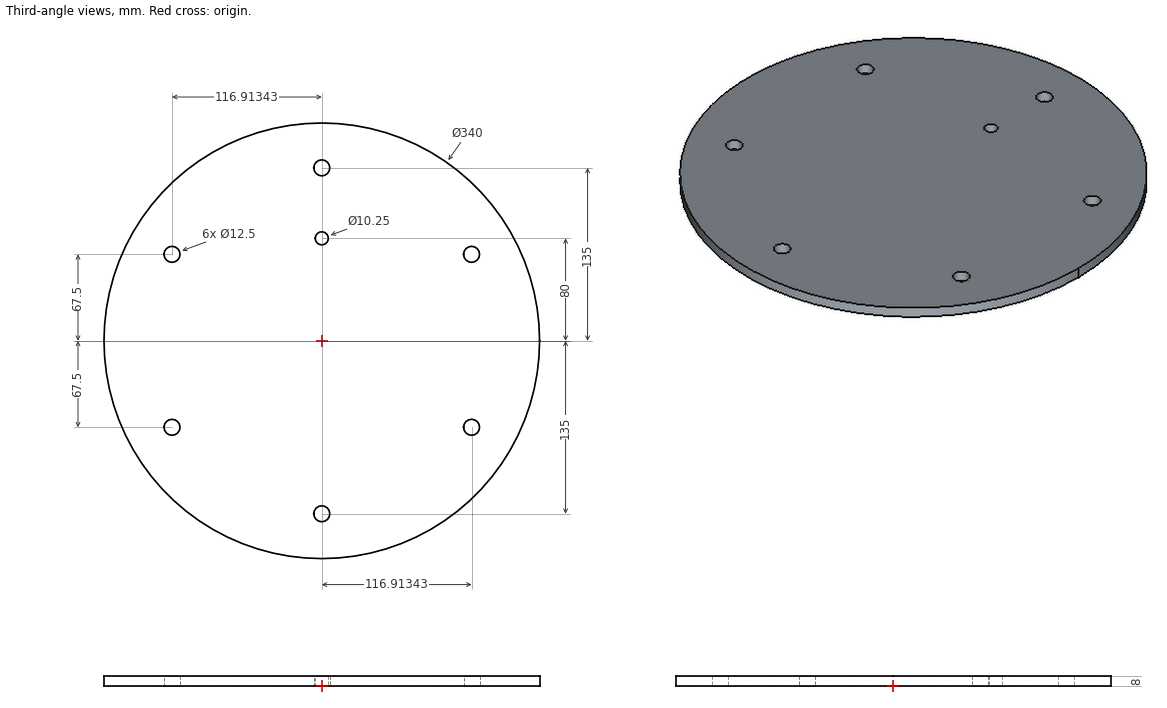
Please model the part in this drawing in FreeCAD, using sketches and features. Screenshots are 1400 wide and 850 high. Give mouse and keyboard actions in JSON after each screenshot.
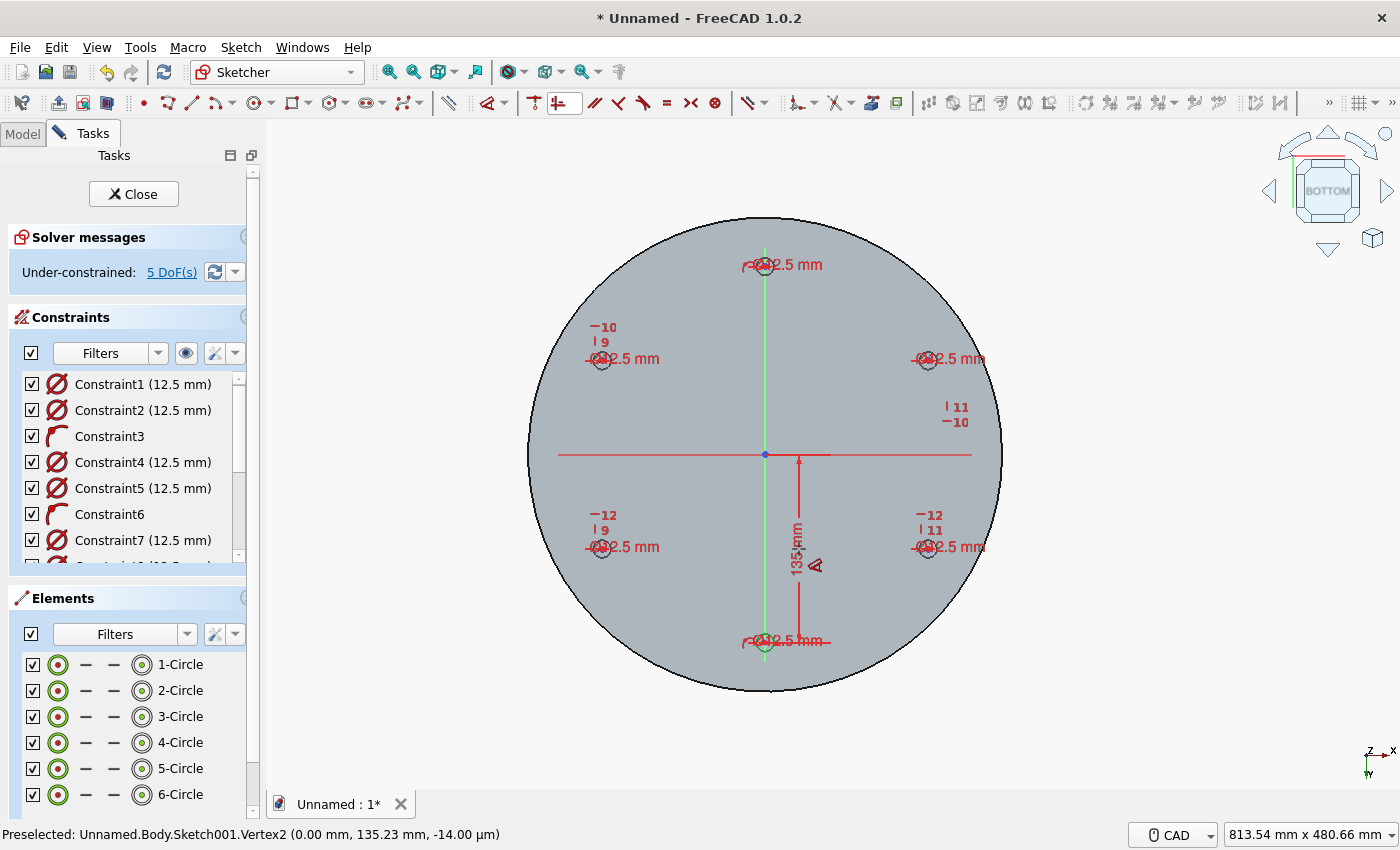
{"action": "left_click", "coordinate": [765, 267]}
{"action": "left_click", "coordinate": [799, 361]}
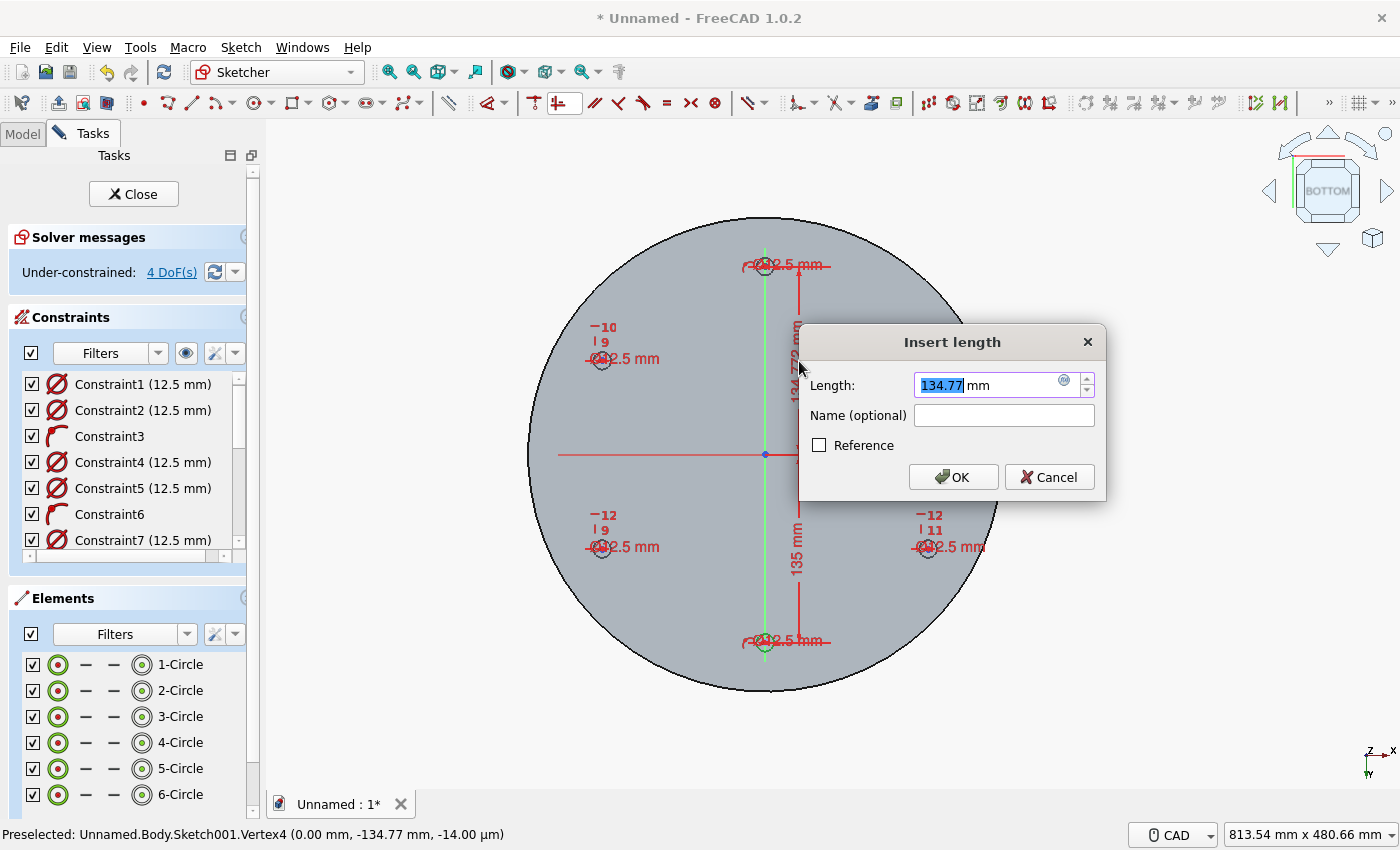
{"action": "type", "text": "135"}
{"action": "key", "text": "Return"}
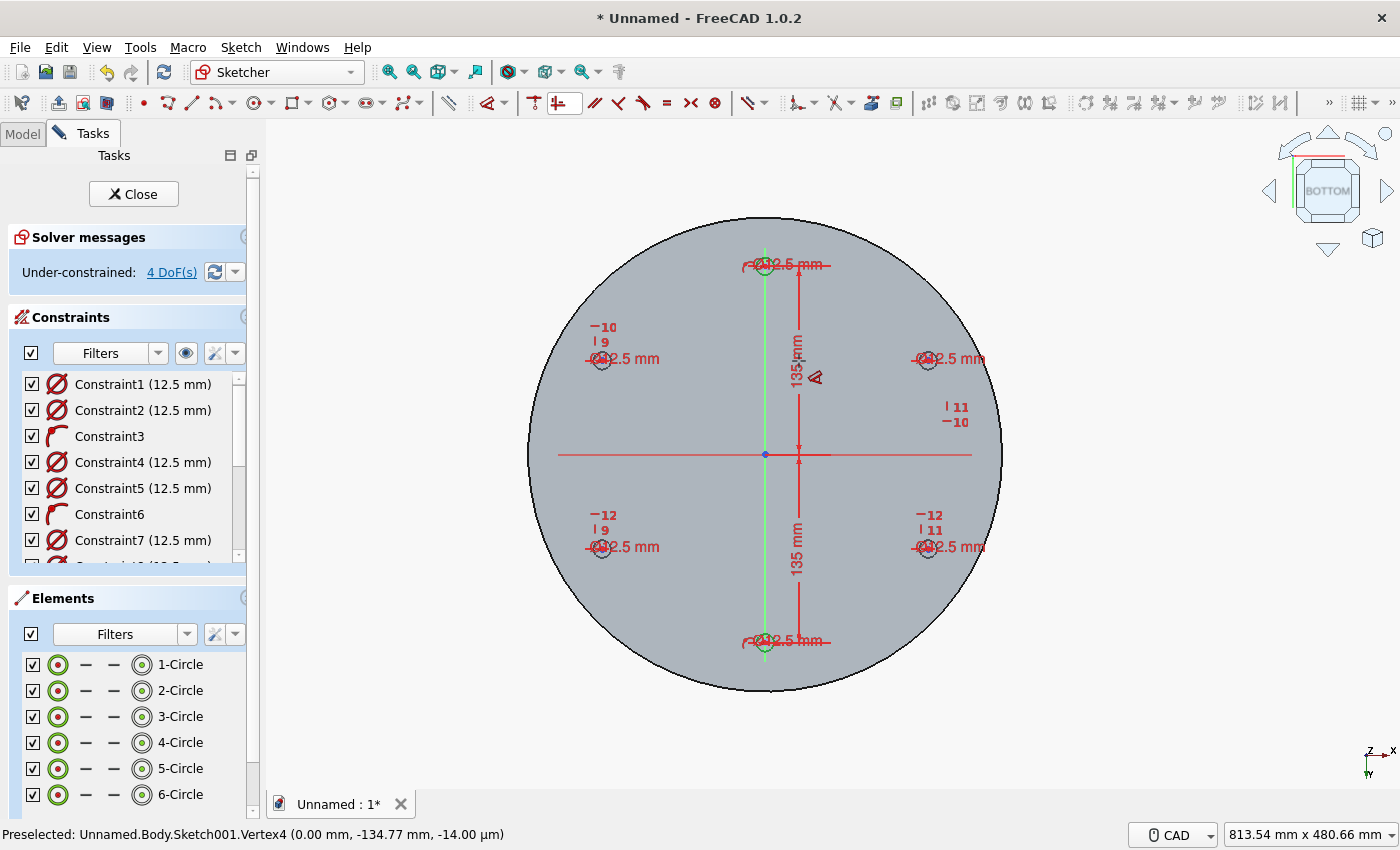
{"action": "left_click", "coordinate": [602, 549]}
{"action": "left_click", "coordinate": [568, 502]}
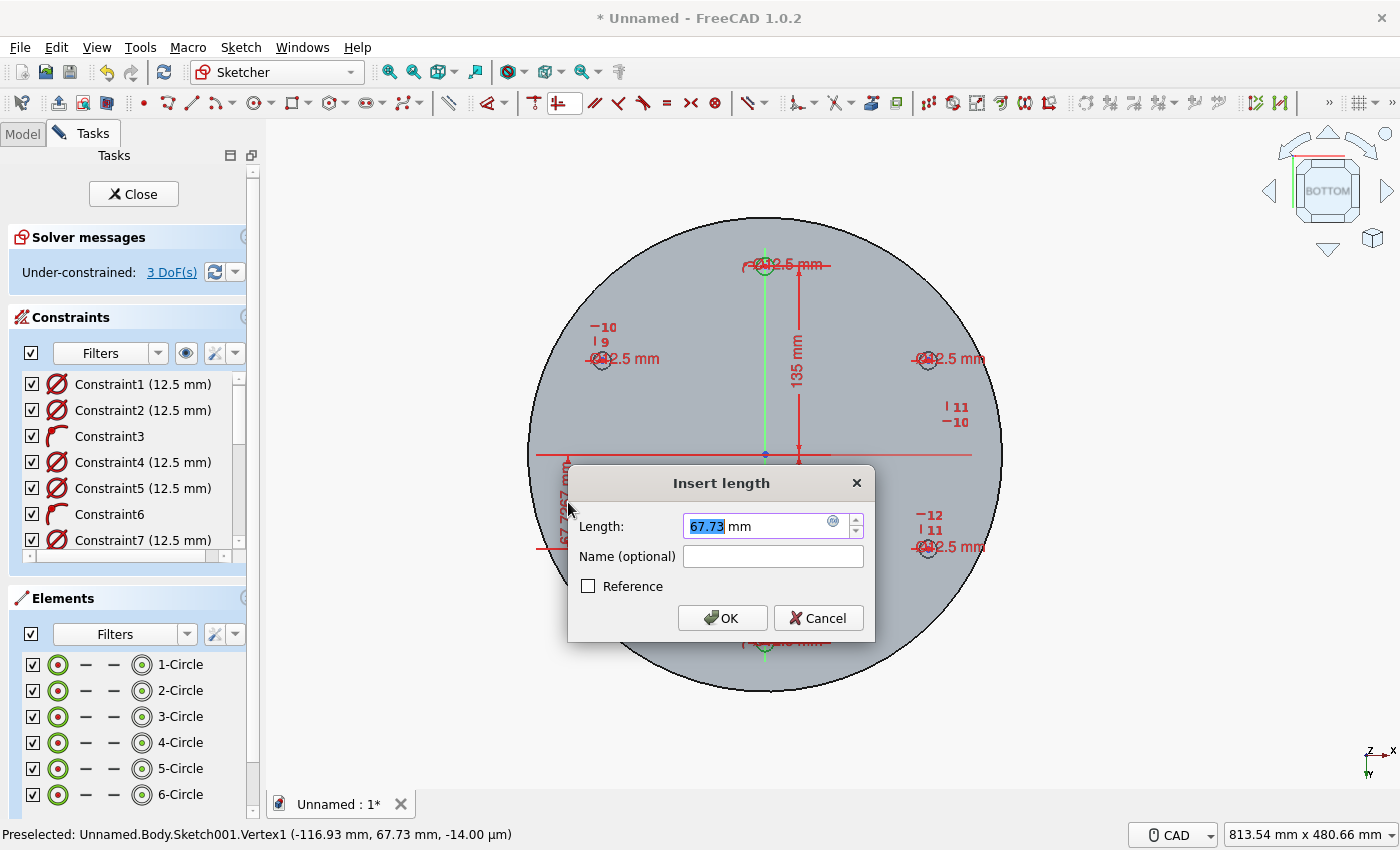
{"action": "type", "text": "67.5"}
{"action": "key", "text": "Return"}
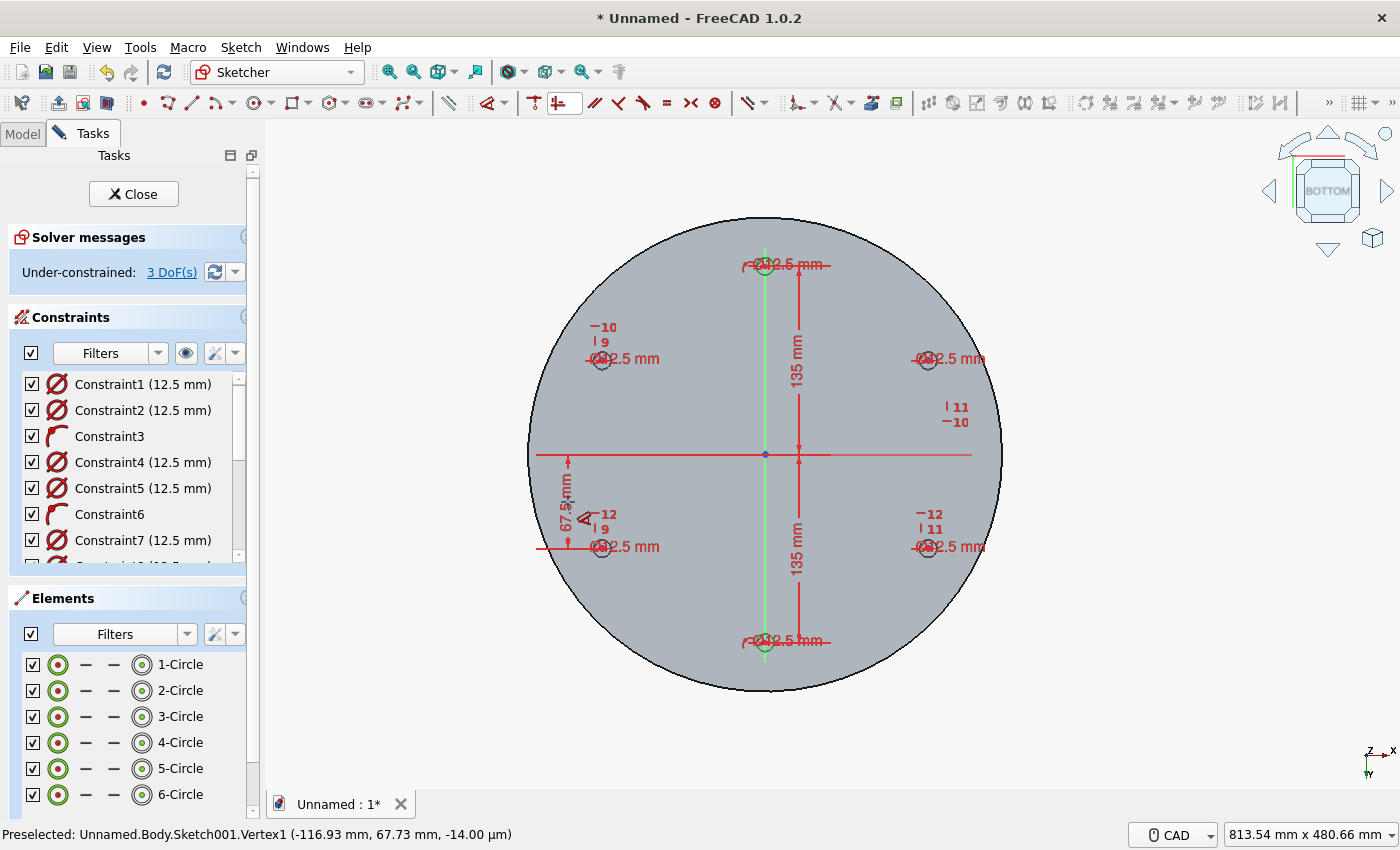
{"action": "left_click", "coordinate": [602, 361]}
{"action": "left_click", "coordinate": [568, 408]}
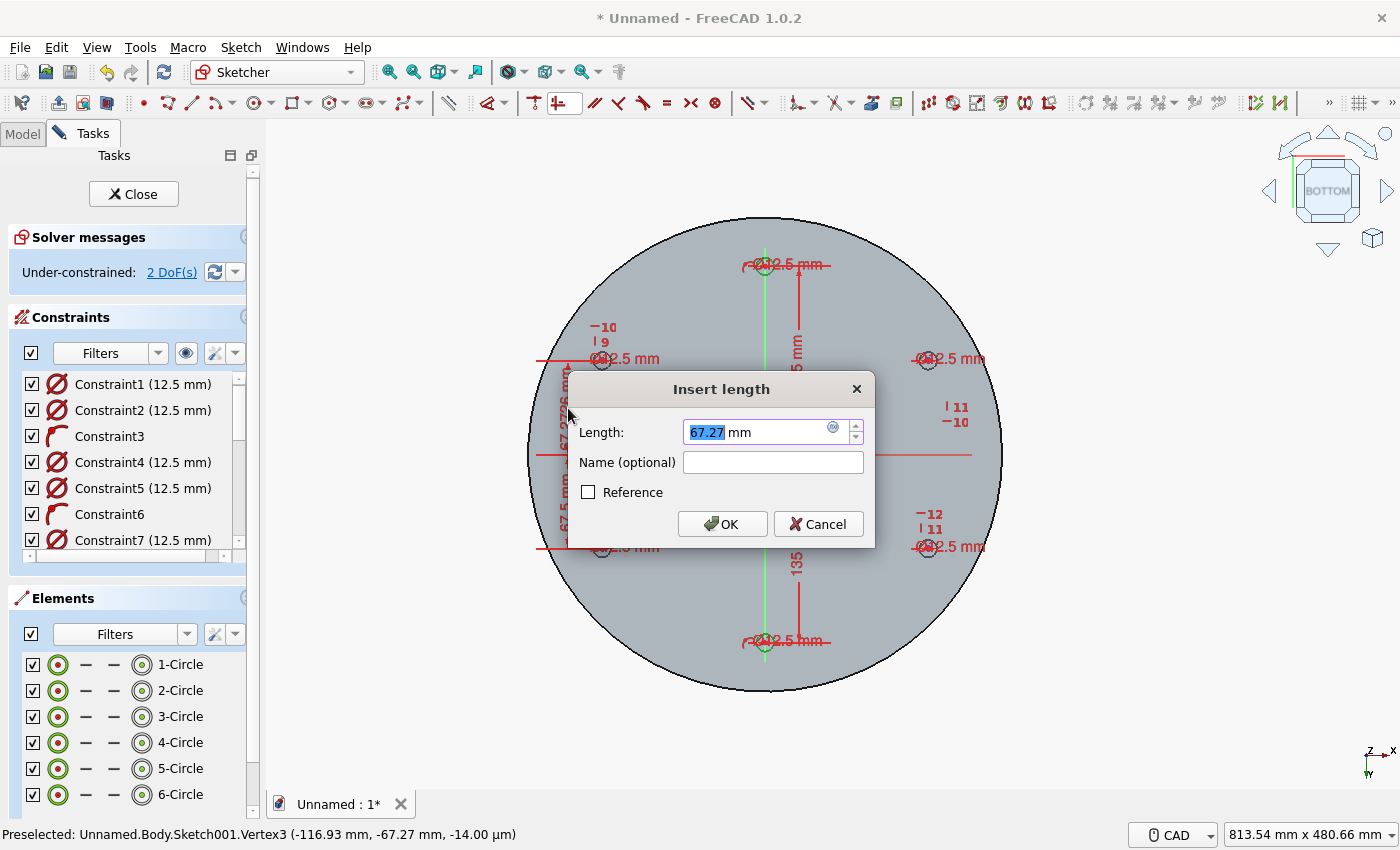
{"action": "type", "text": "67.5"}
{"action": "key", "text": "Return"}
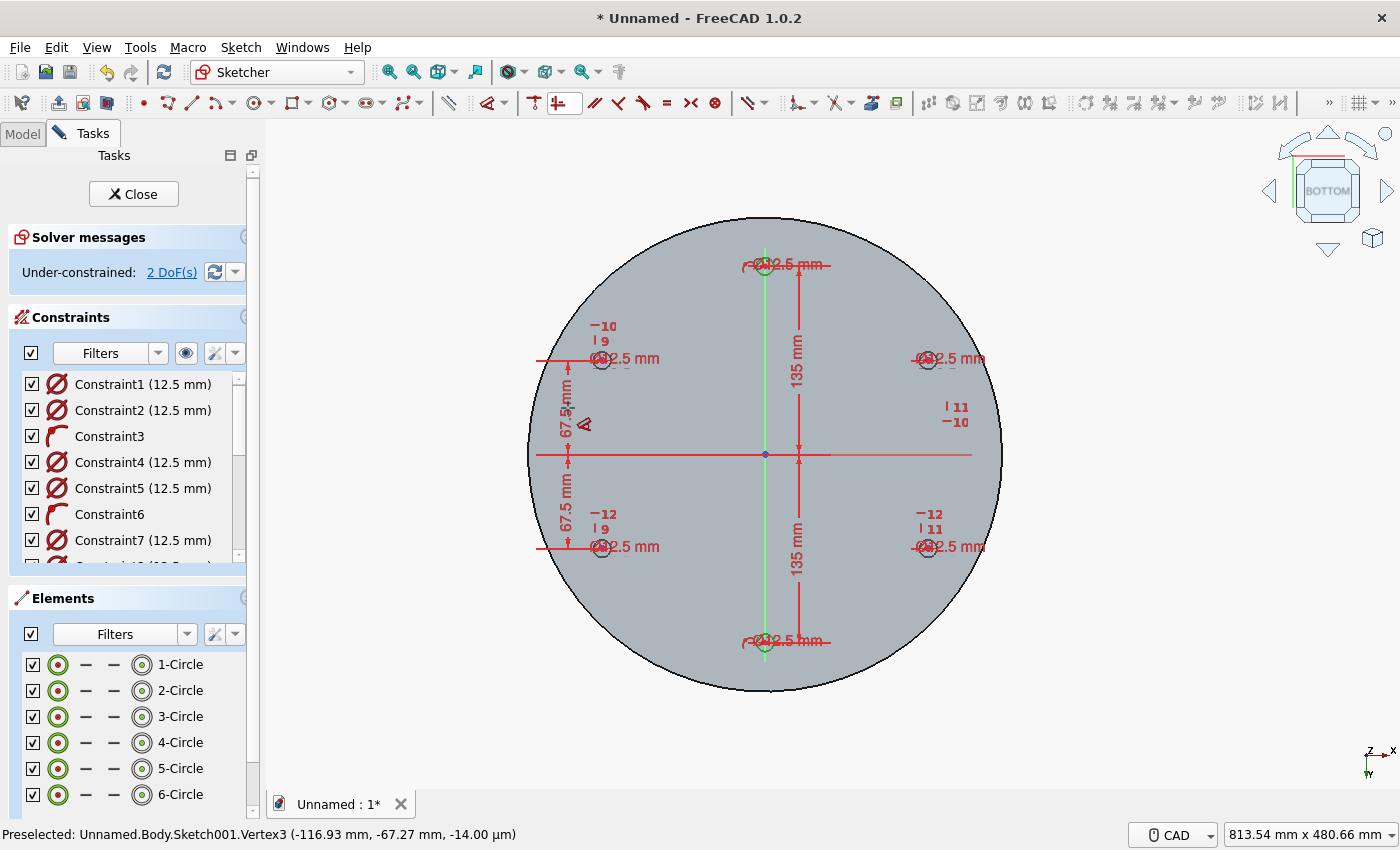
{"action": "left_click", "coordinate": [602, 549]}
{"action": "left_click", "coordinate": [684, 583]}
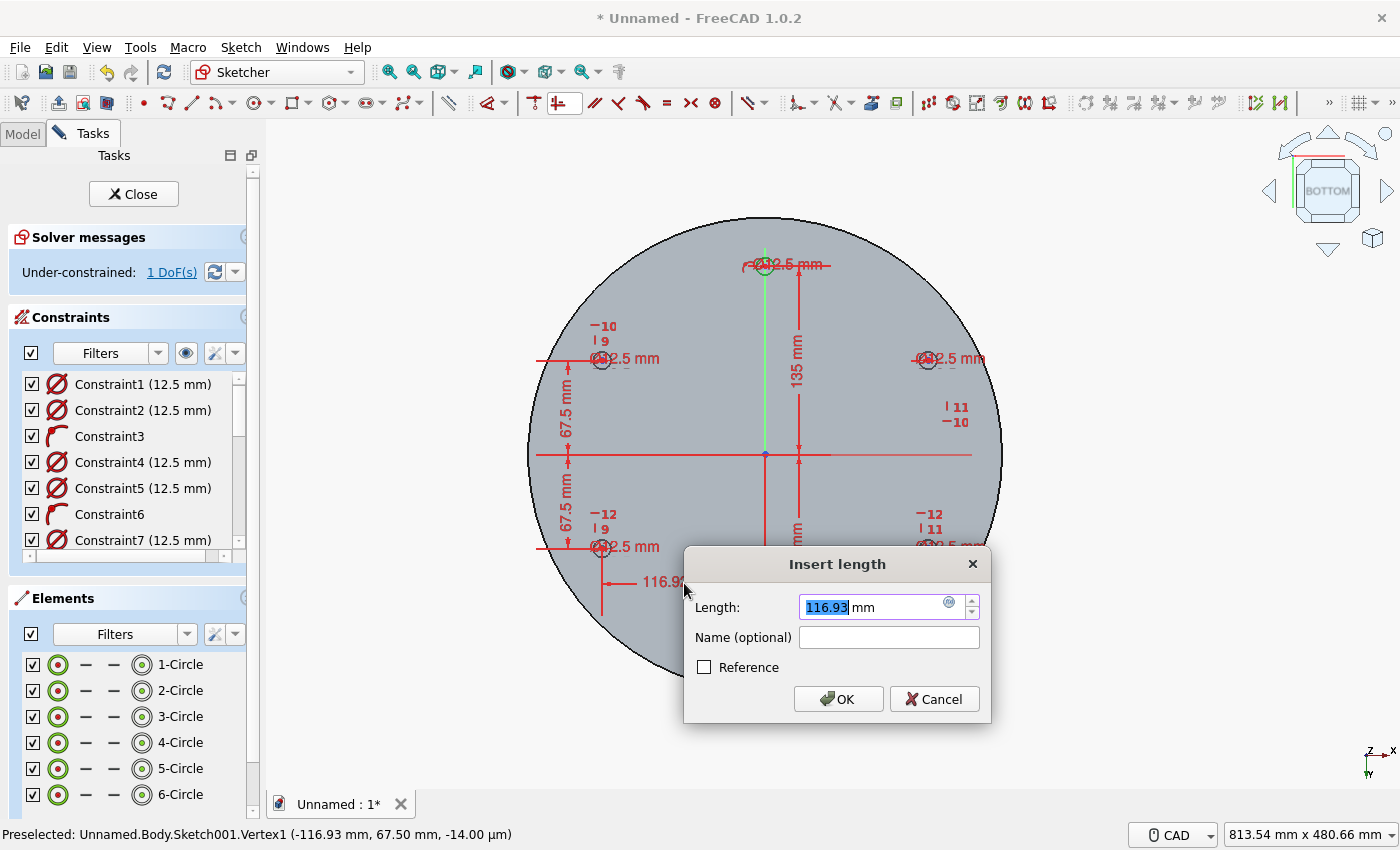
{"action": "type", "text": "116.91343"}
{"action": "key", "text": "Return"}